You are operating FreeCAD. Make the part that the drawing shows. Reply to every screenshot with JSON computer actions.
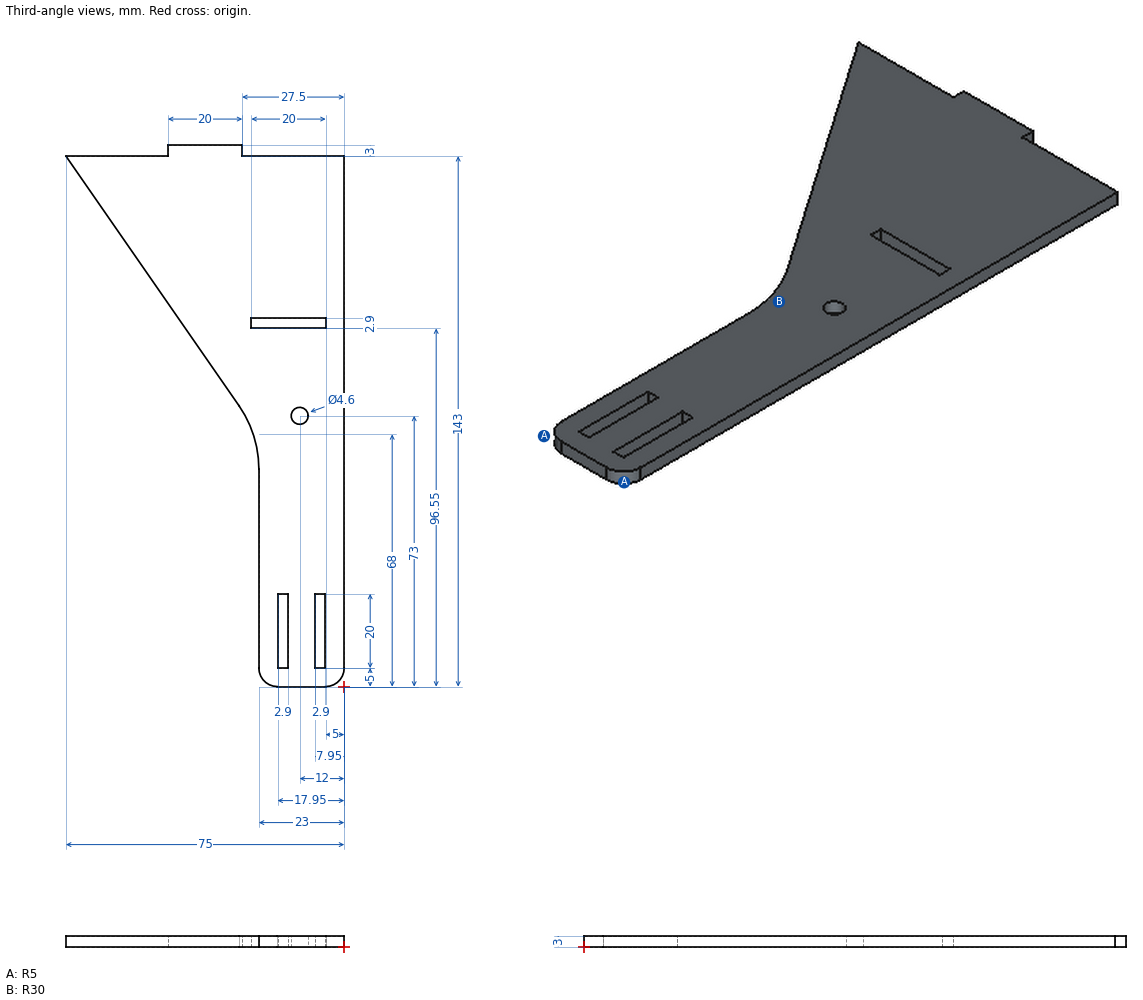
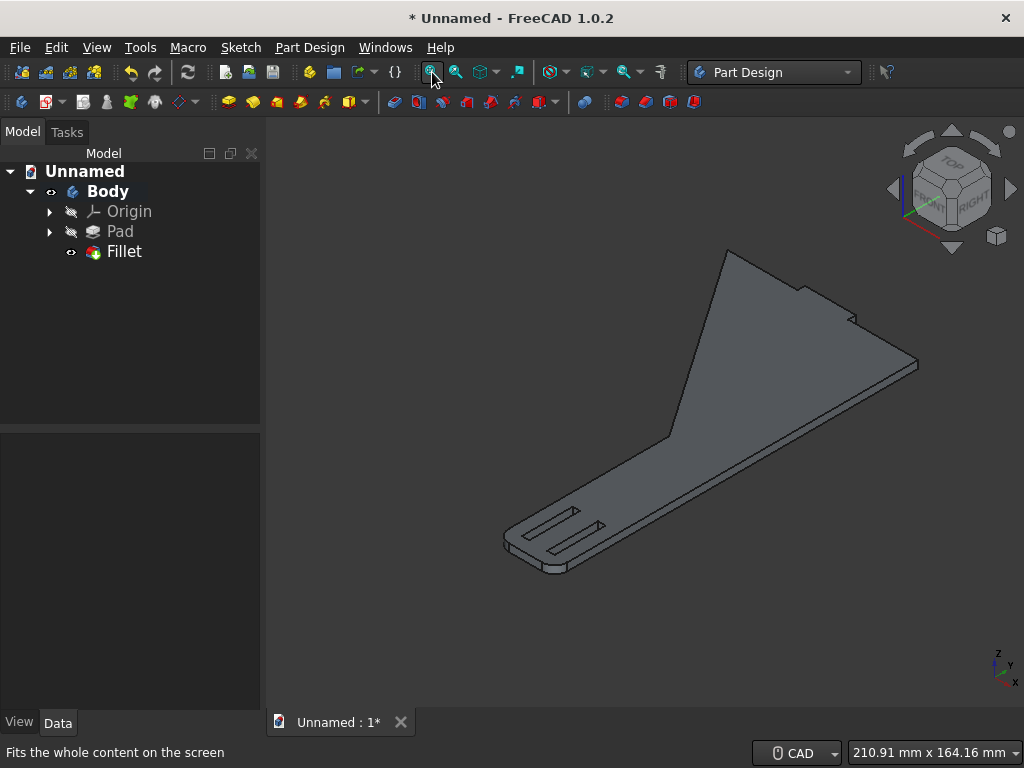
{"action": "key", "text": "2"}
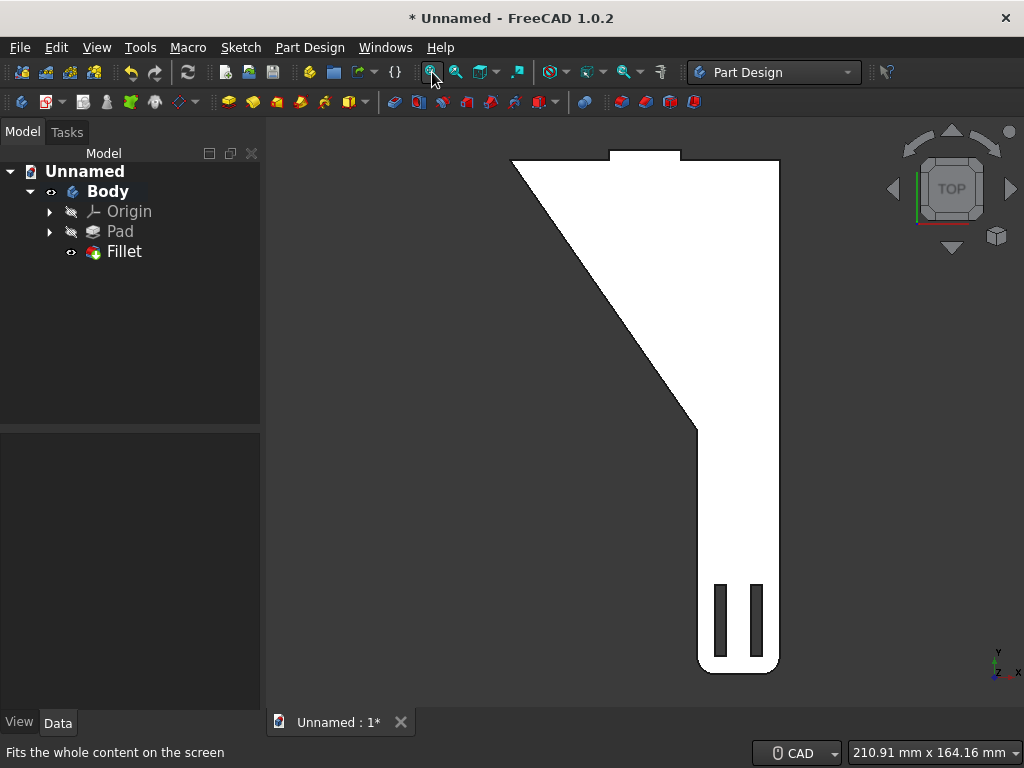
{"action": "scroll", "coordinate": [697, 429], "scroll_direction": "up", "scroll_amount": 7}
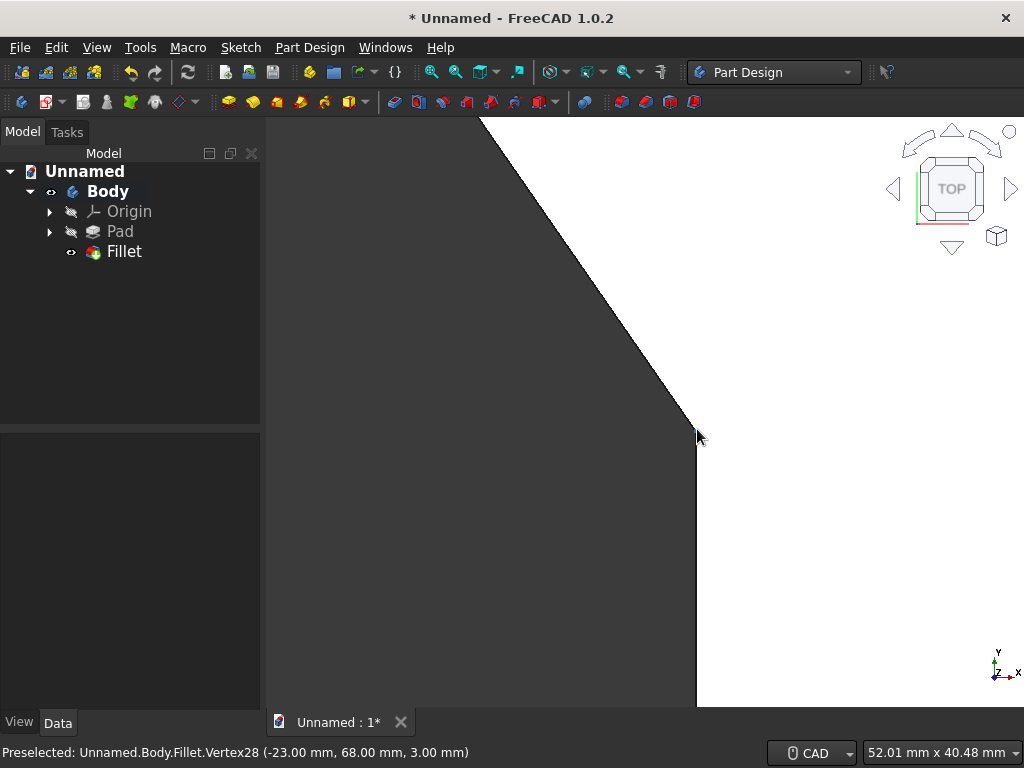
{"action": "left_click", "coordinate": [432, 72]}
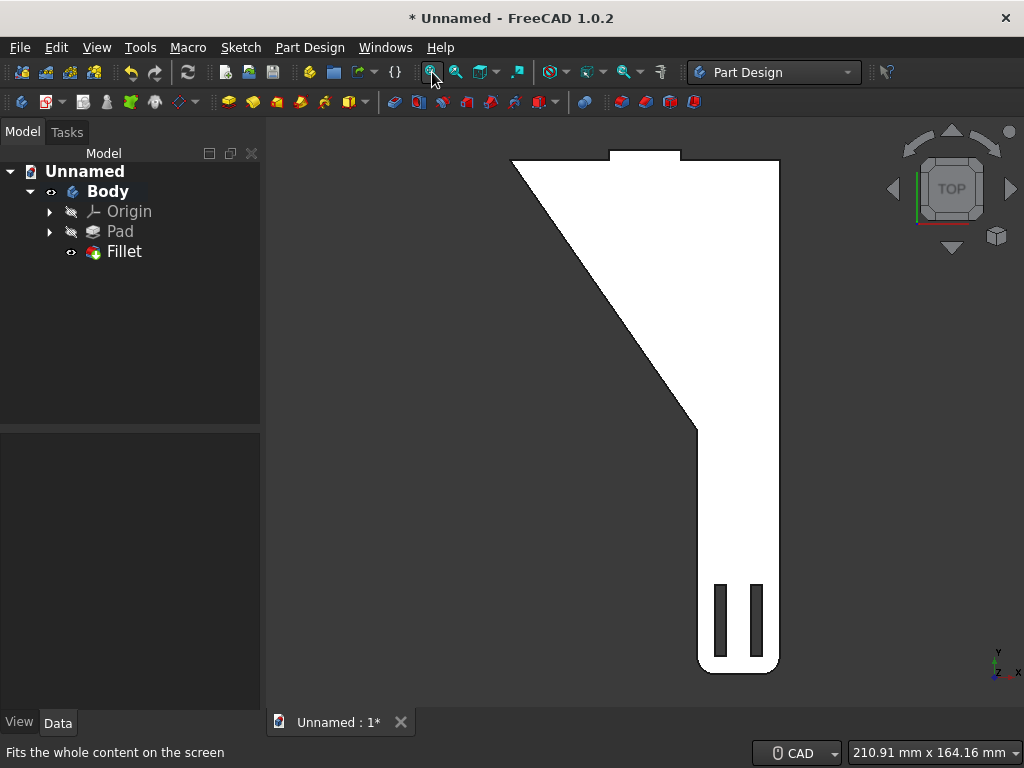
{"action": "key", "text": "1"}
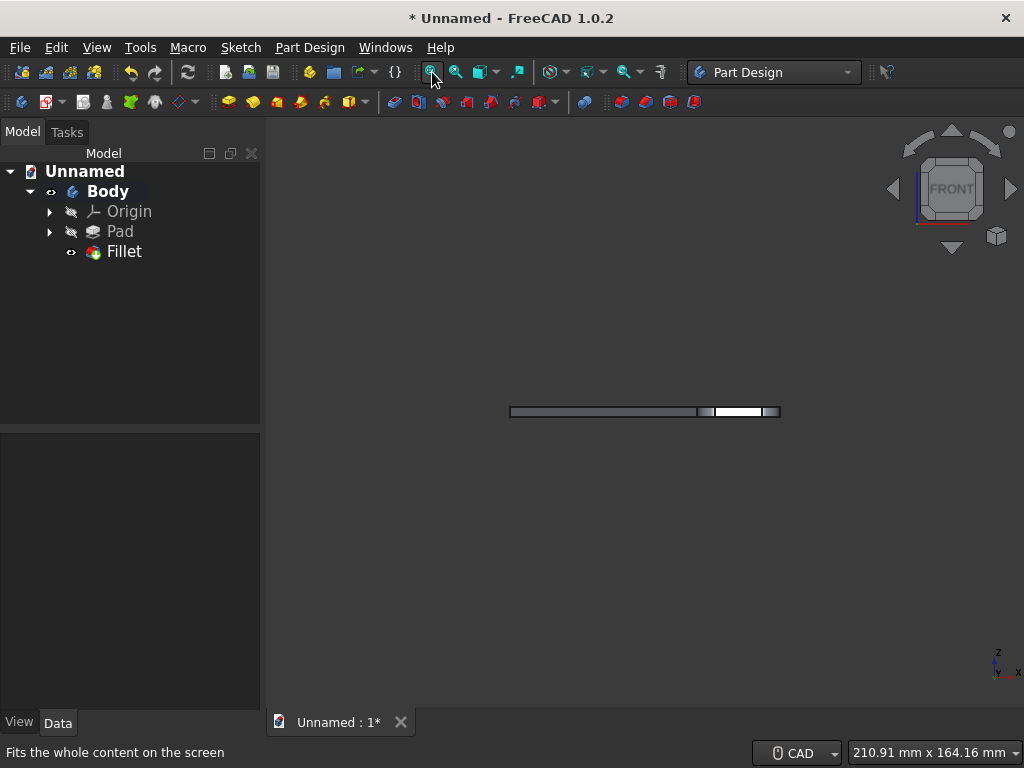
{"action": "left_click", "coordinate": [432, 72]}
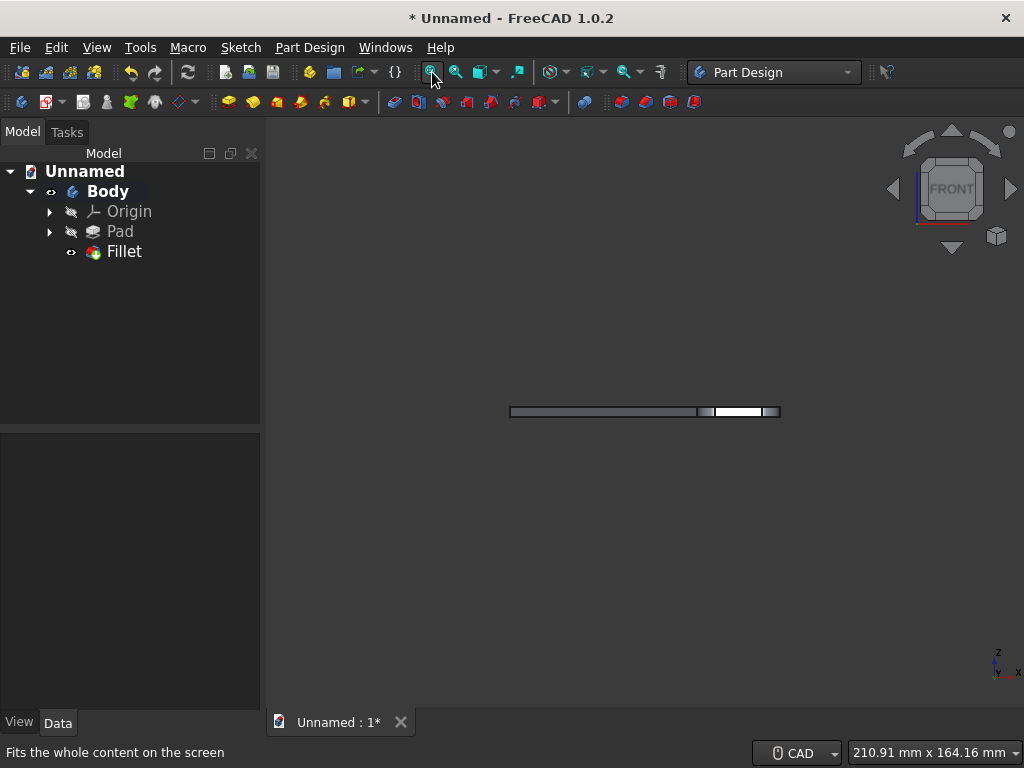
{"action": "scroll", "coordinate": [697, 411], "scroll_direction": "up", "scroll_amount": 7}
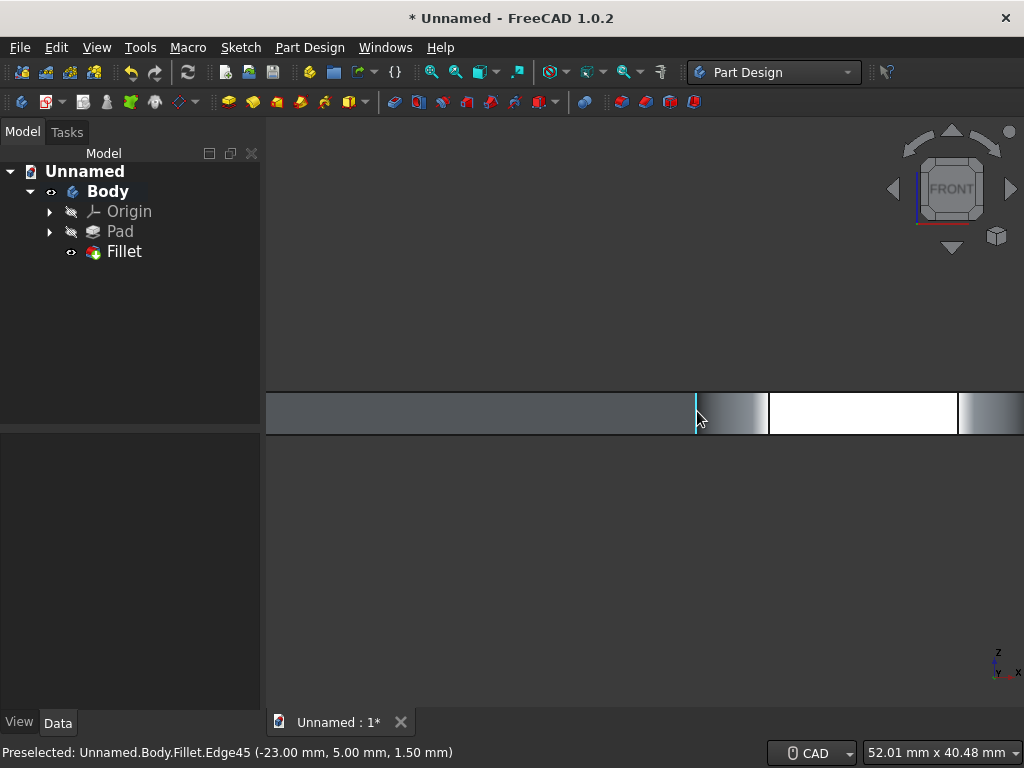
{"action": "left_click", "coordinate": [432, 72]}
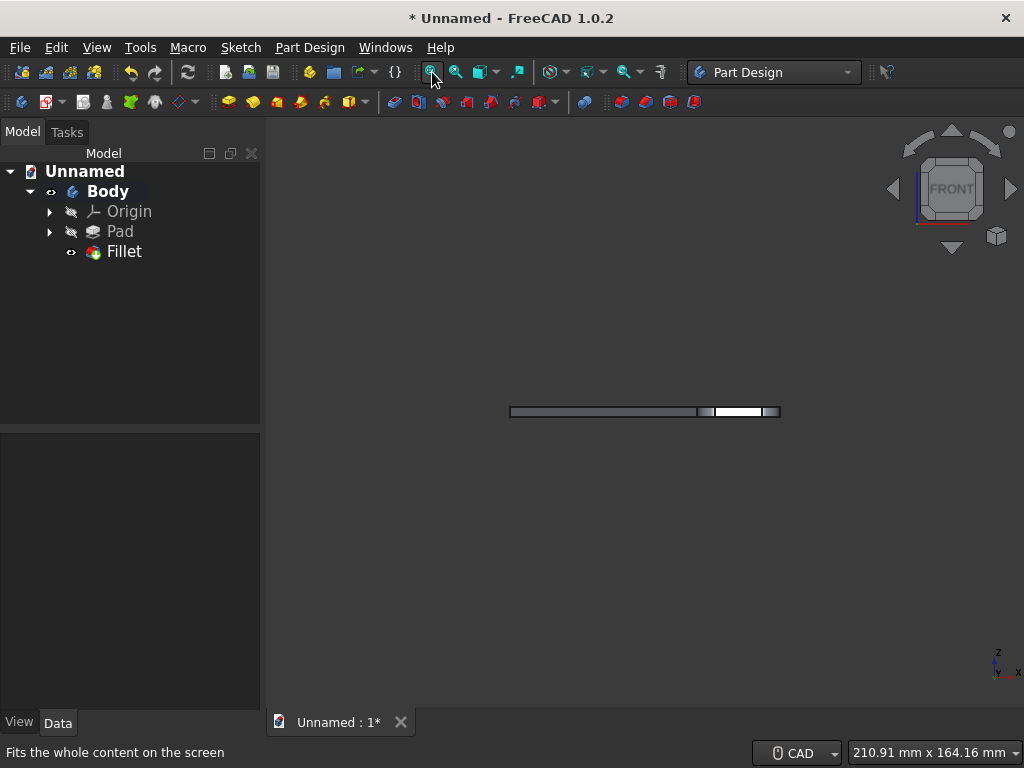
{"action": "key", "text": "3"}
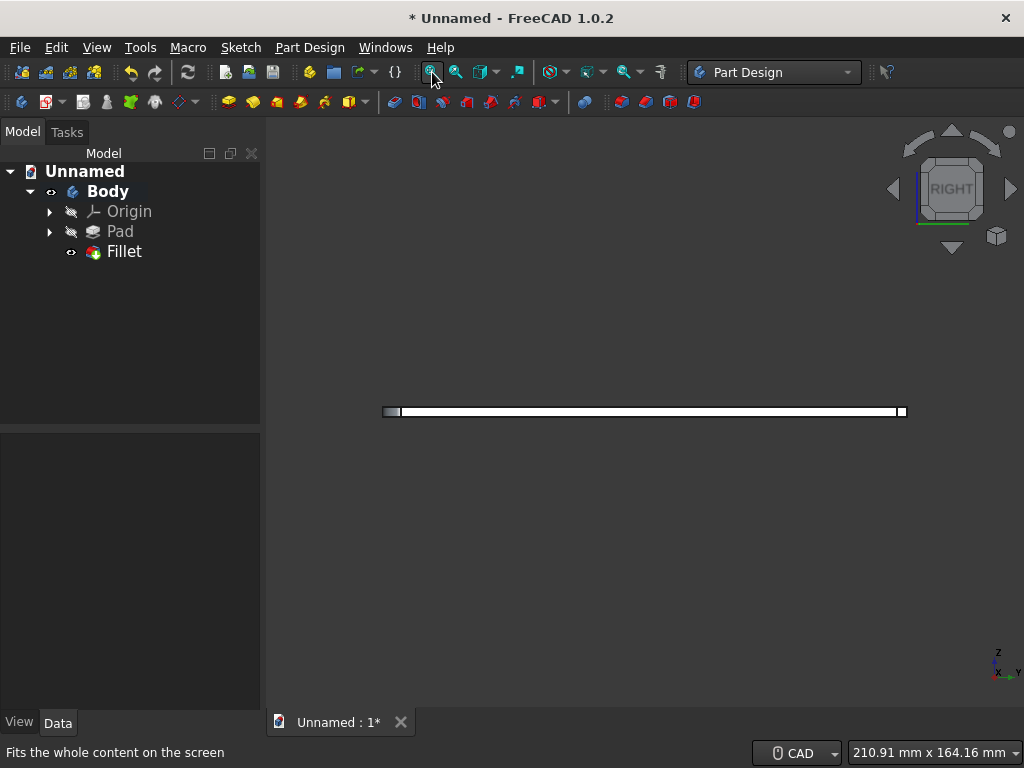
{"action": "scroll", "coordinate": [627, 411], "scroll_direction": "up", "scroll_amount": 7}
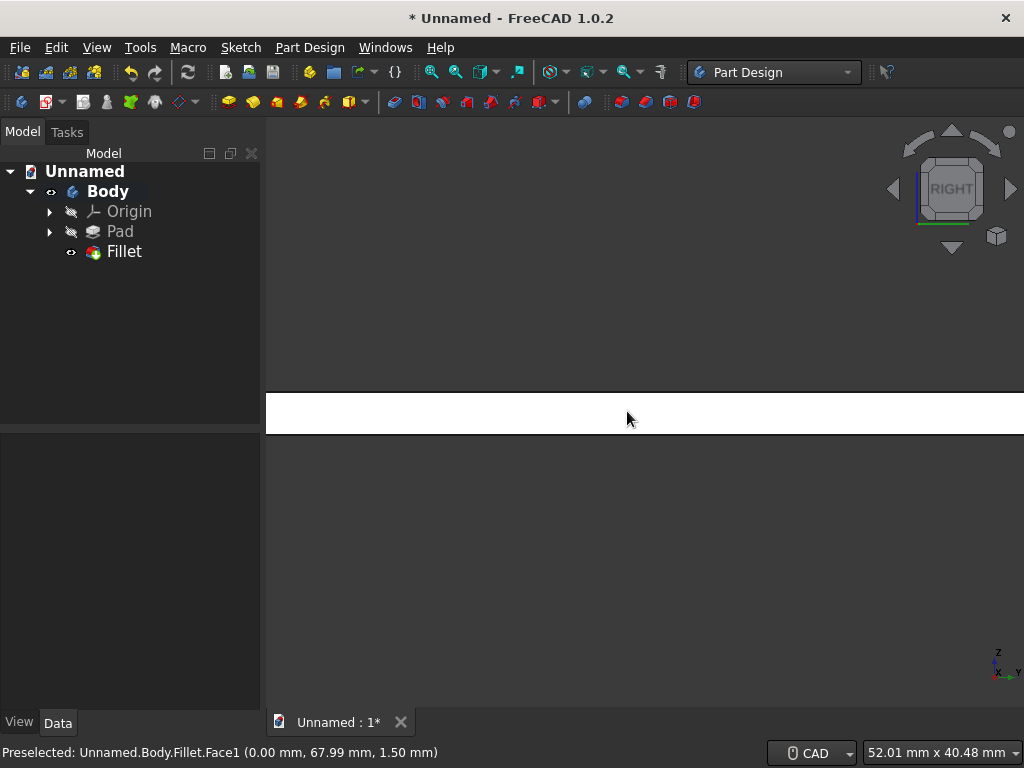
{"action": "left_click", "coordinate": [432, 72]}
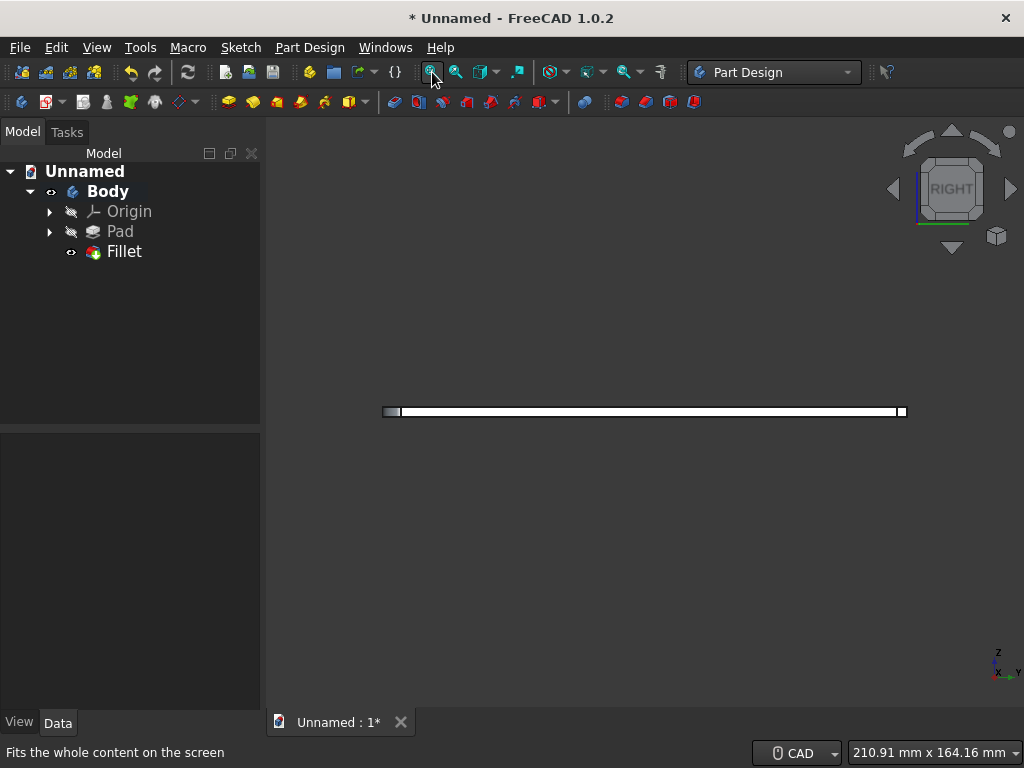
{"action": "key", "text": "5"}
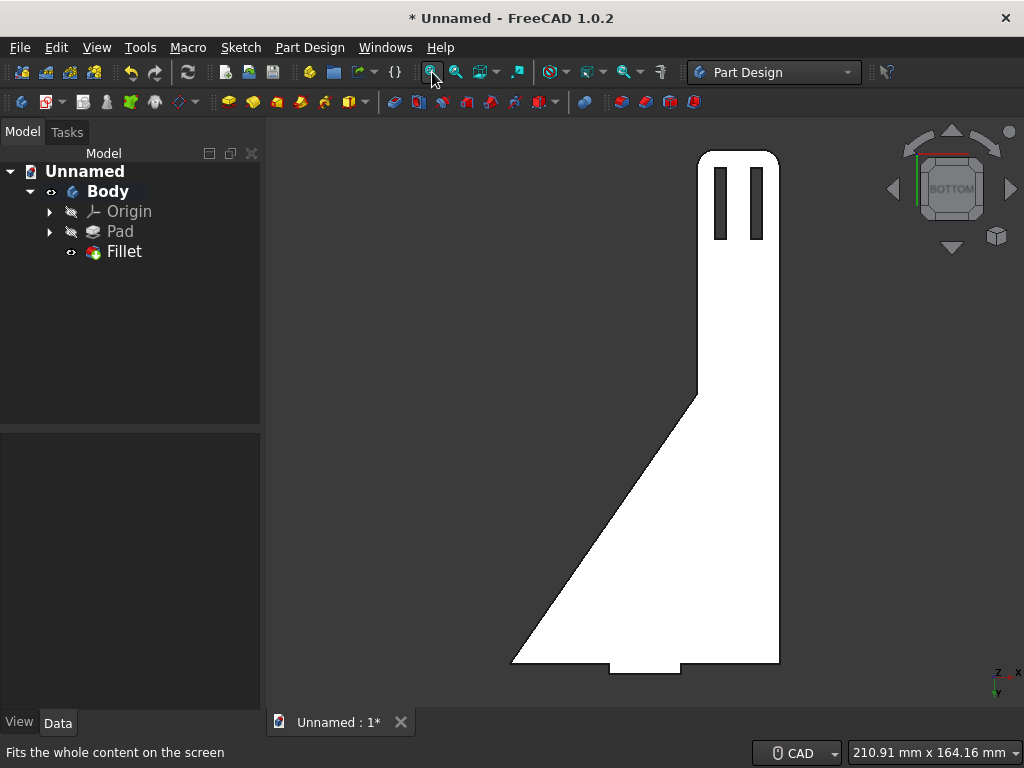
{"action": "scroll", "coordinate": [697, 393], "scroll_direction": "up", "scroll_amount": 7}